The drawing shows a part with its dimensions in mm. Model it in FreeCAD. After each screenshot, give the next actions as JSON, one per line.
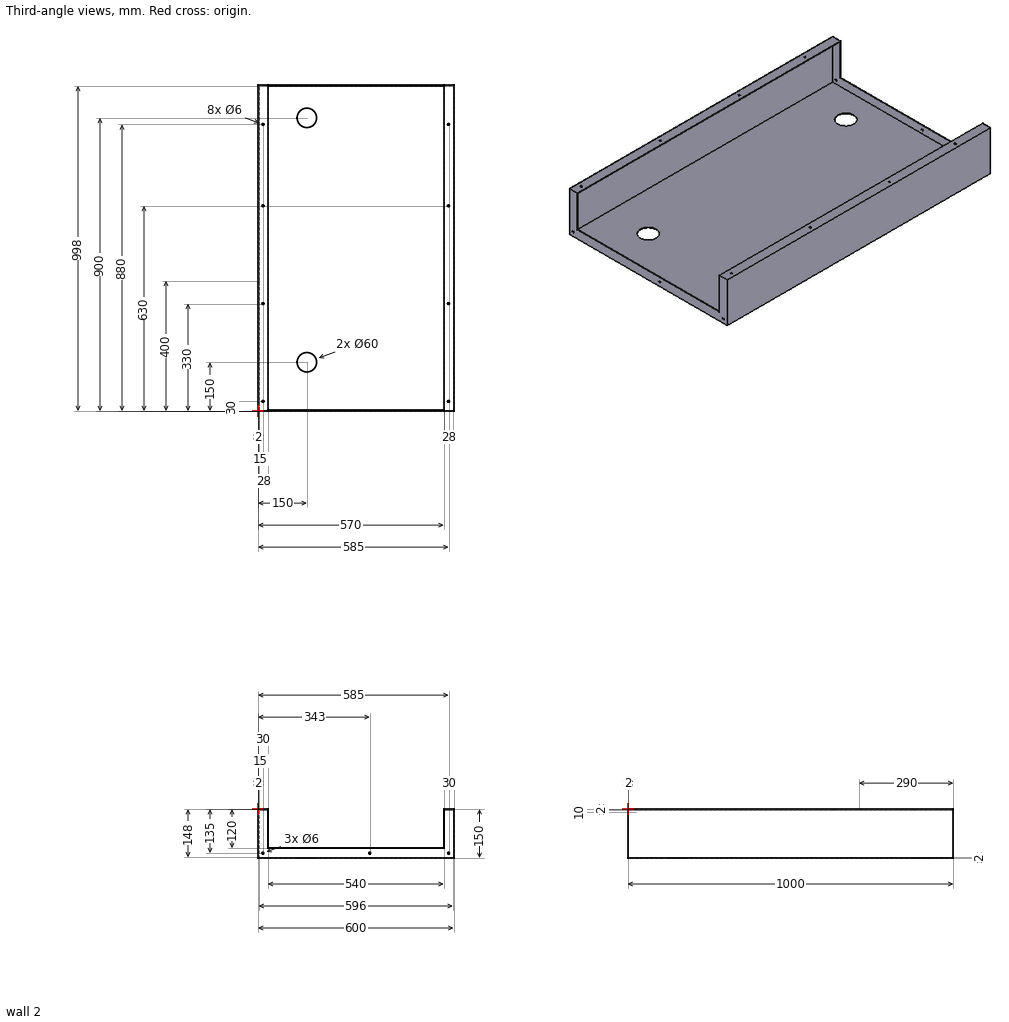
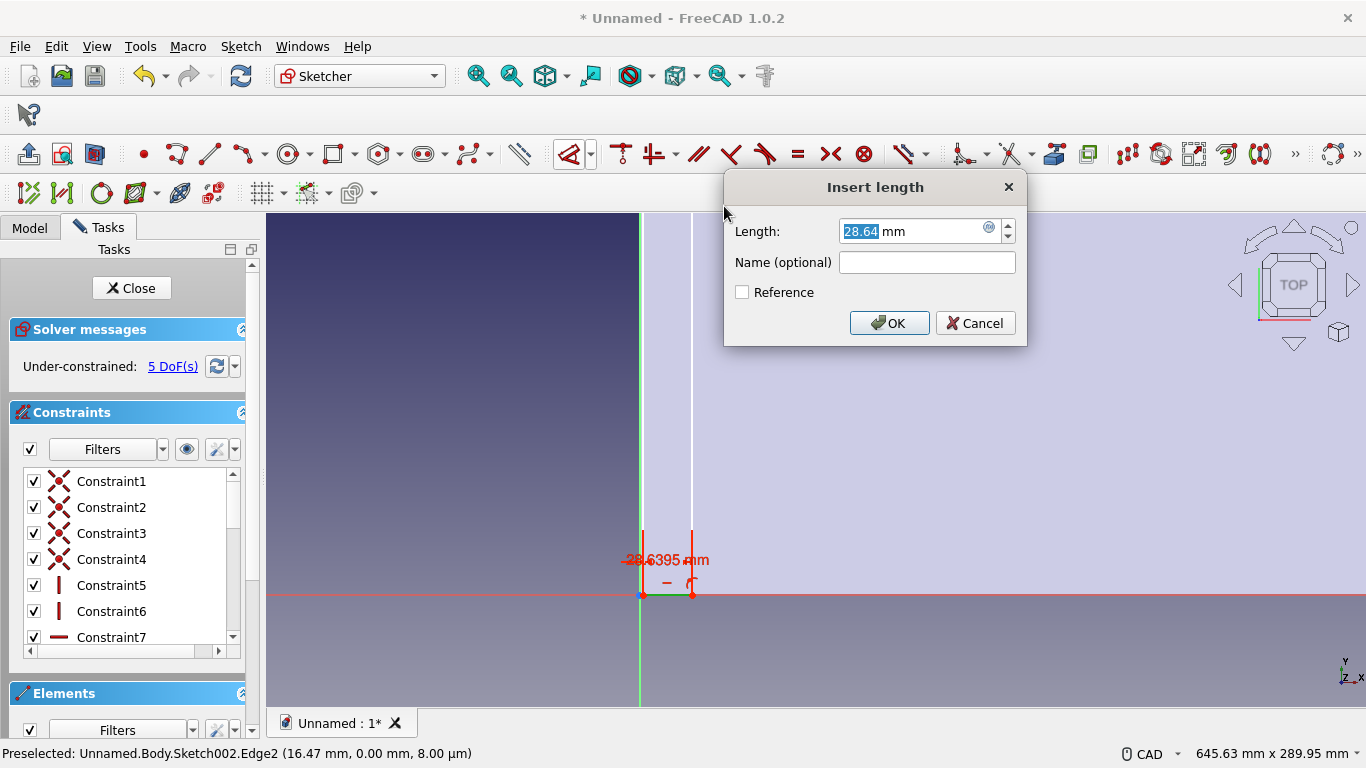
{"action": "type", "text": "28"}
{"action": "key", "text": "Return"}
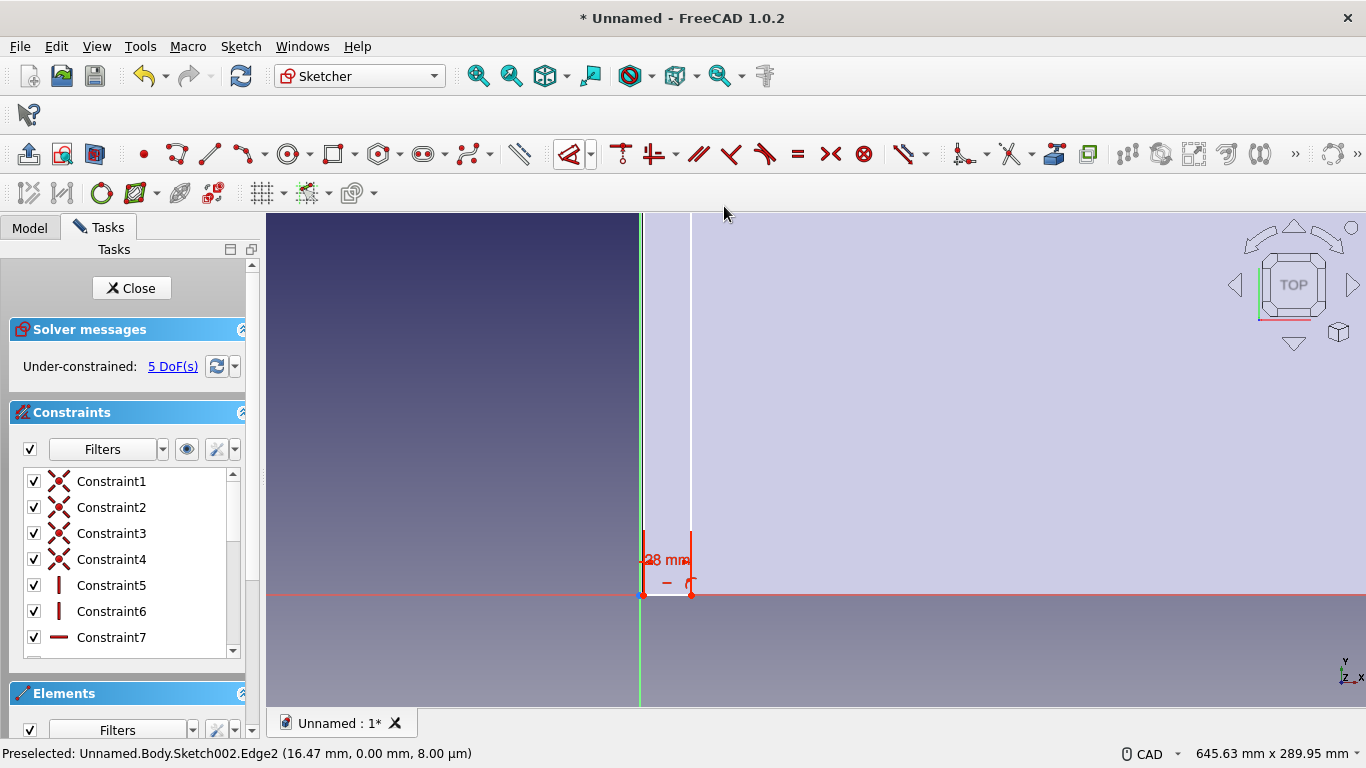
{"action": "scroll", "coordinate": [668, 602], "scroll_direction": "down", "scroll_amount": 9}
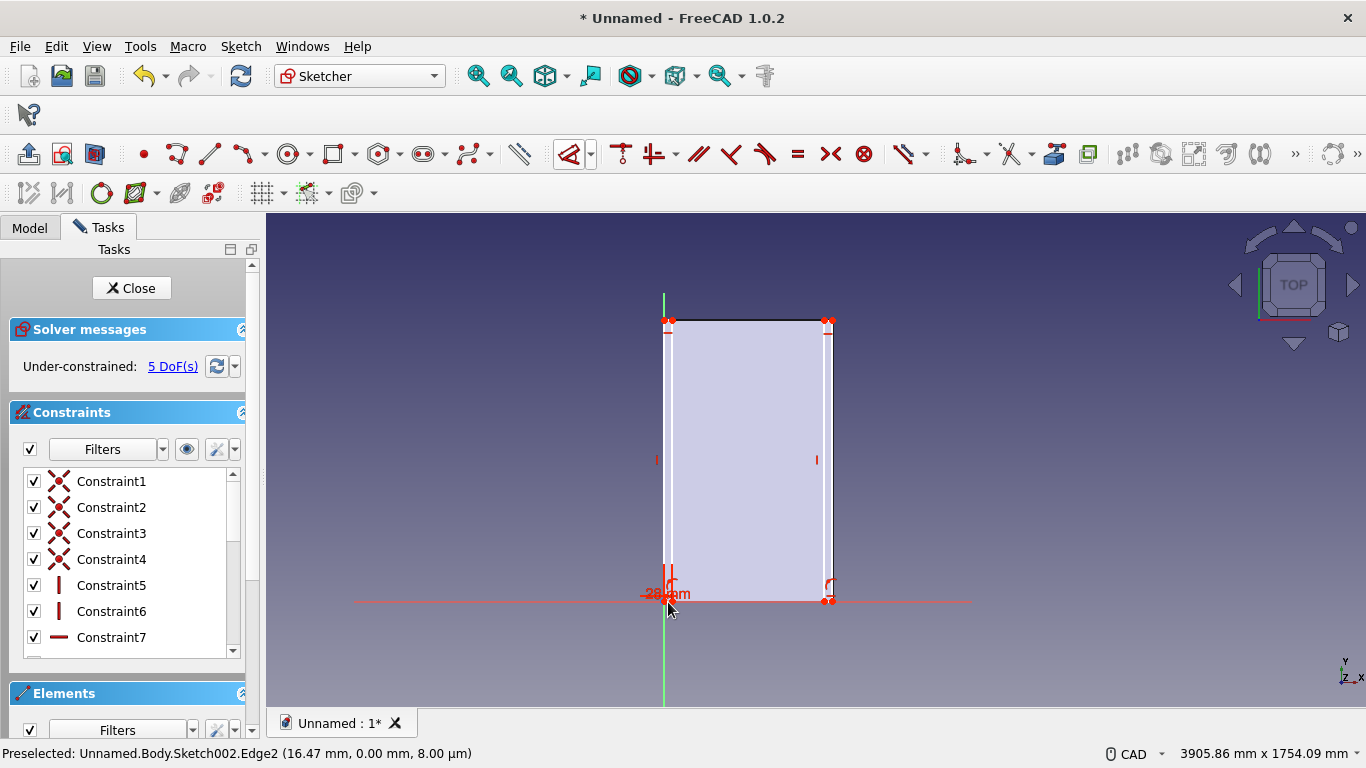
{"action": "scroll", "coordinate": [827, 602], "scroll_direction": "up", "scroll_amount": 9}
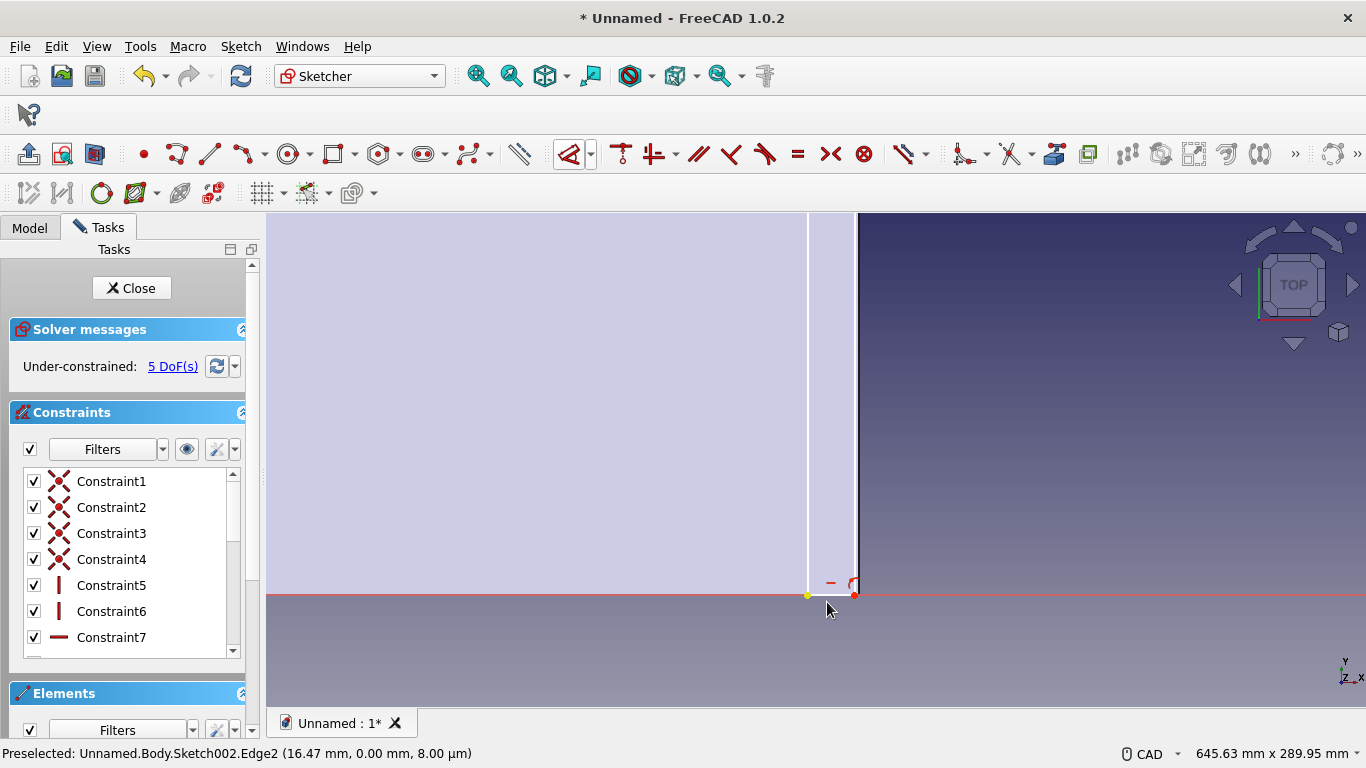
{"action": "left_click", "coordinate": [822, 595]}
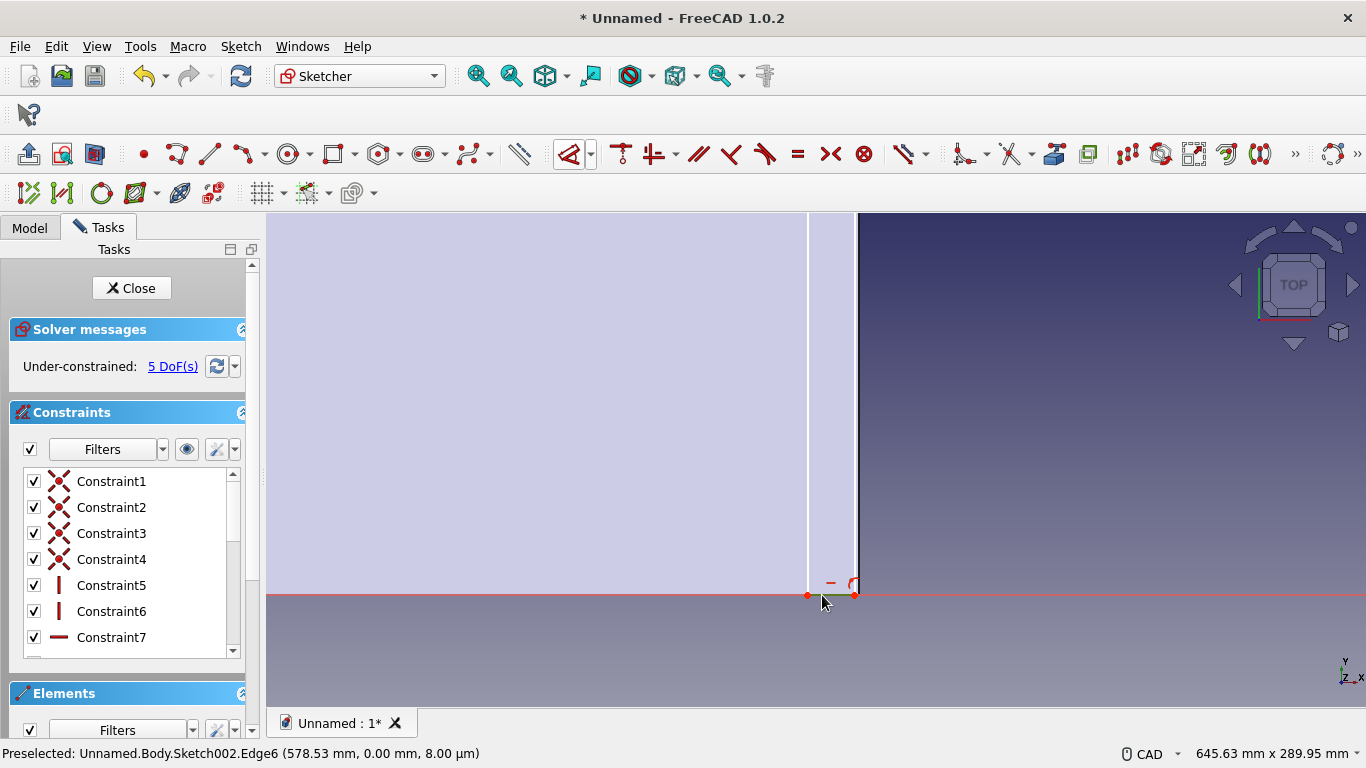
{"action": "left_click", "coordinate": [590, 154]}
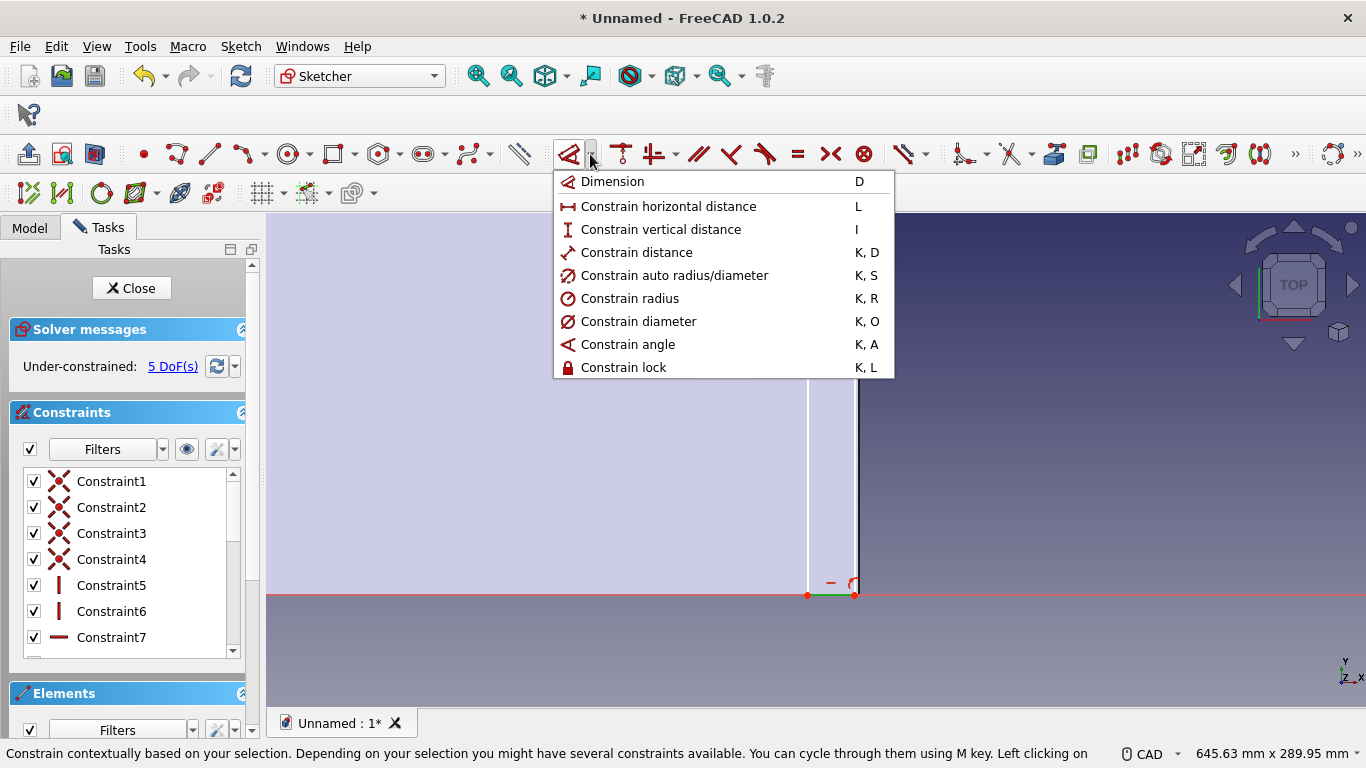
{"action": "left_click", "coordinate": [724, 206]}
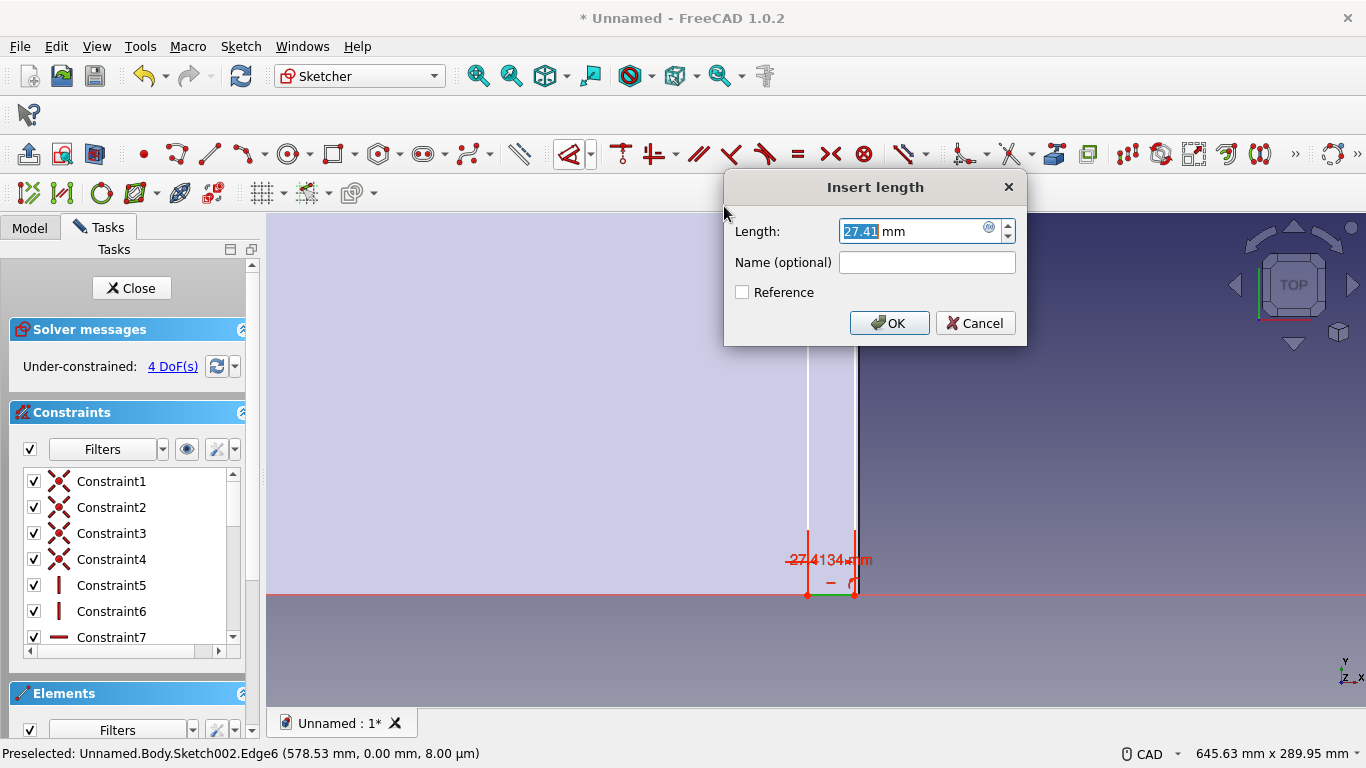
{"action": "type", "text": "28"}
{"action": "key", "text": "Return"}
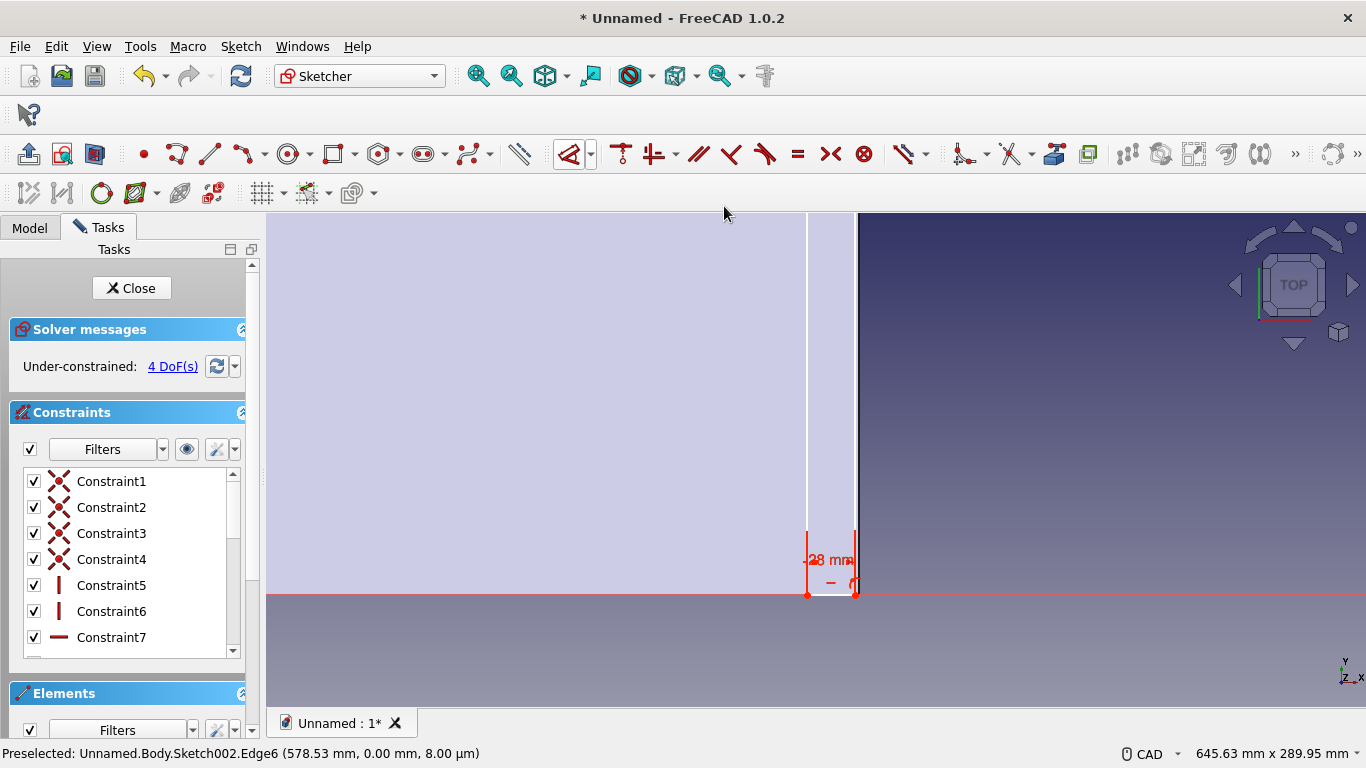
{"action": "scroll", "coordinate": [827, 602], "scroll_direction": "down", "scroll_amount": 9}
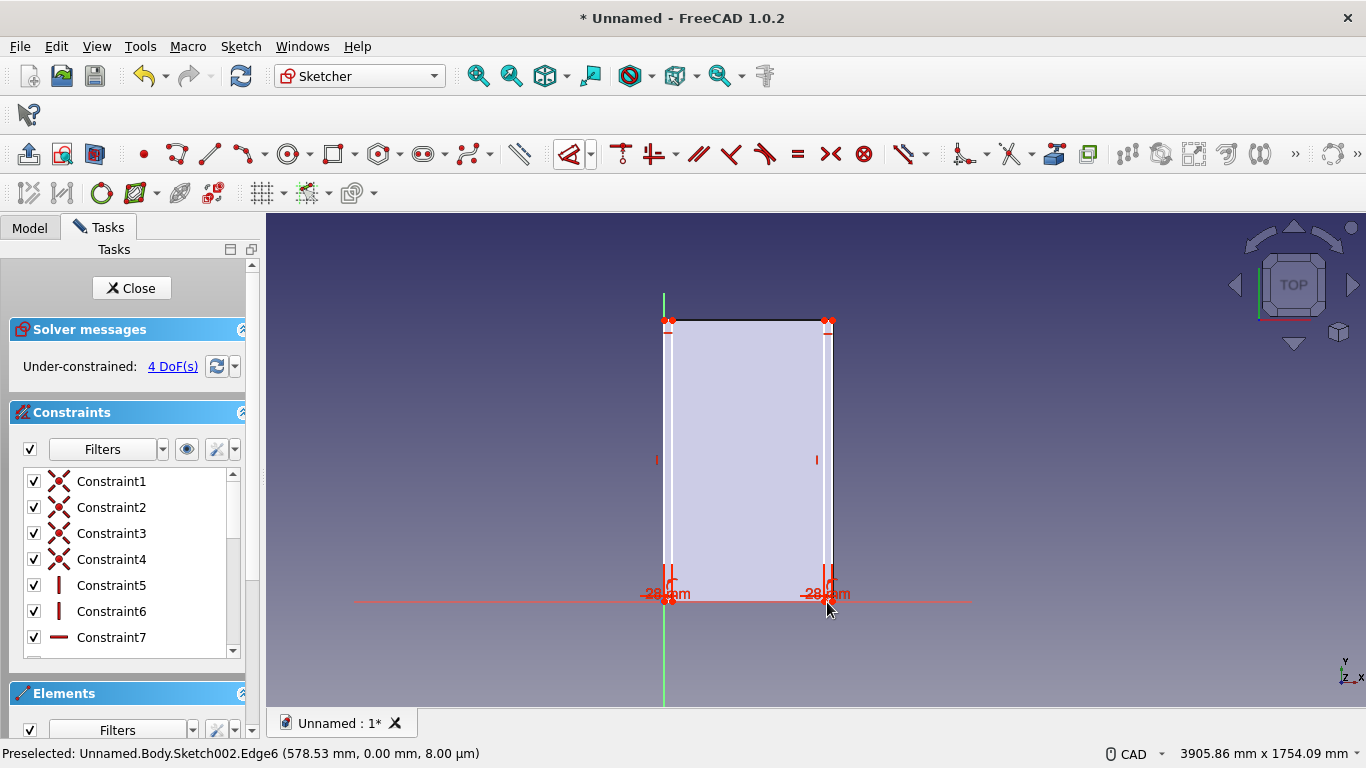
{"action": "scroll", "coordinate": [664, 320], "scroll_direction": "up", "scroll_amount": 22}